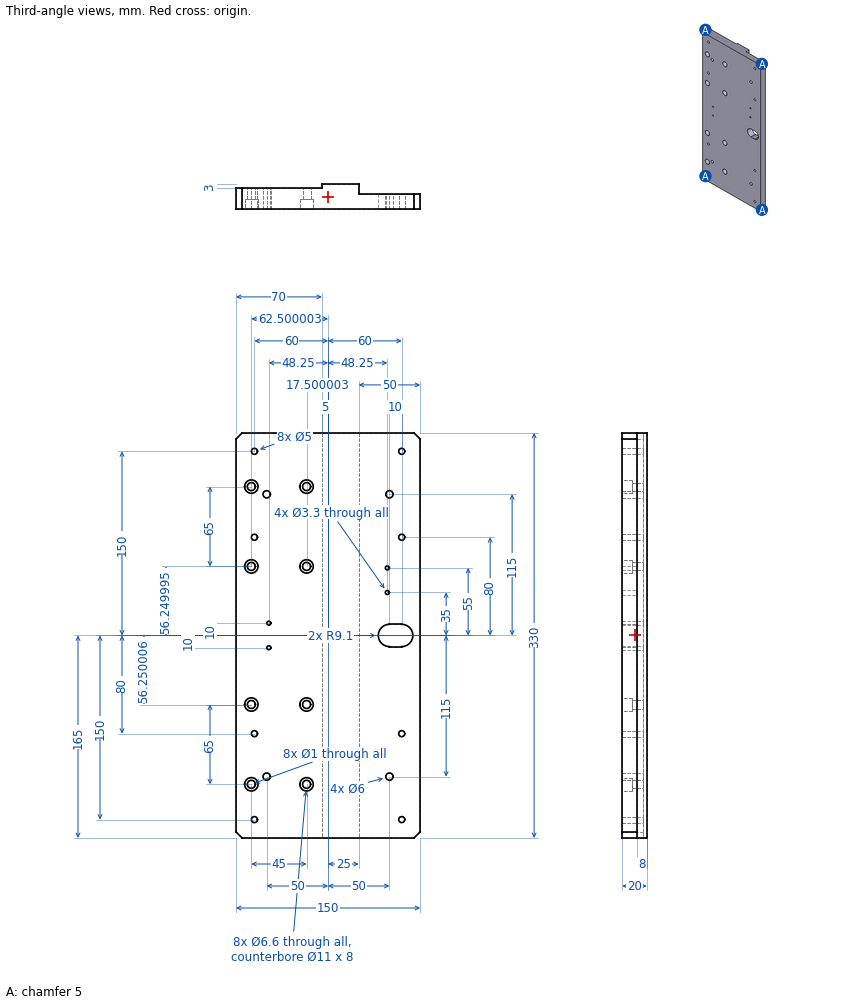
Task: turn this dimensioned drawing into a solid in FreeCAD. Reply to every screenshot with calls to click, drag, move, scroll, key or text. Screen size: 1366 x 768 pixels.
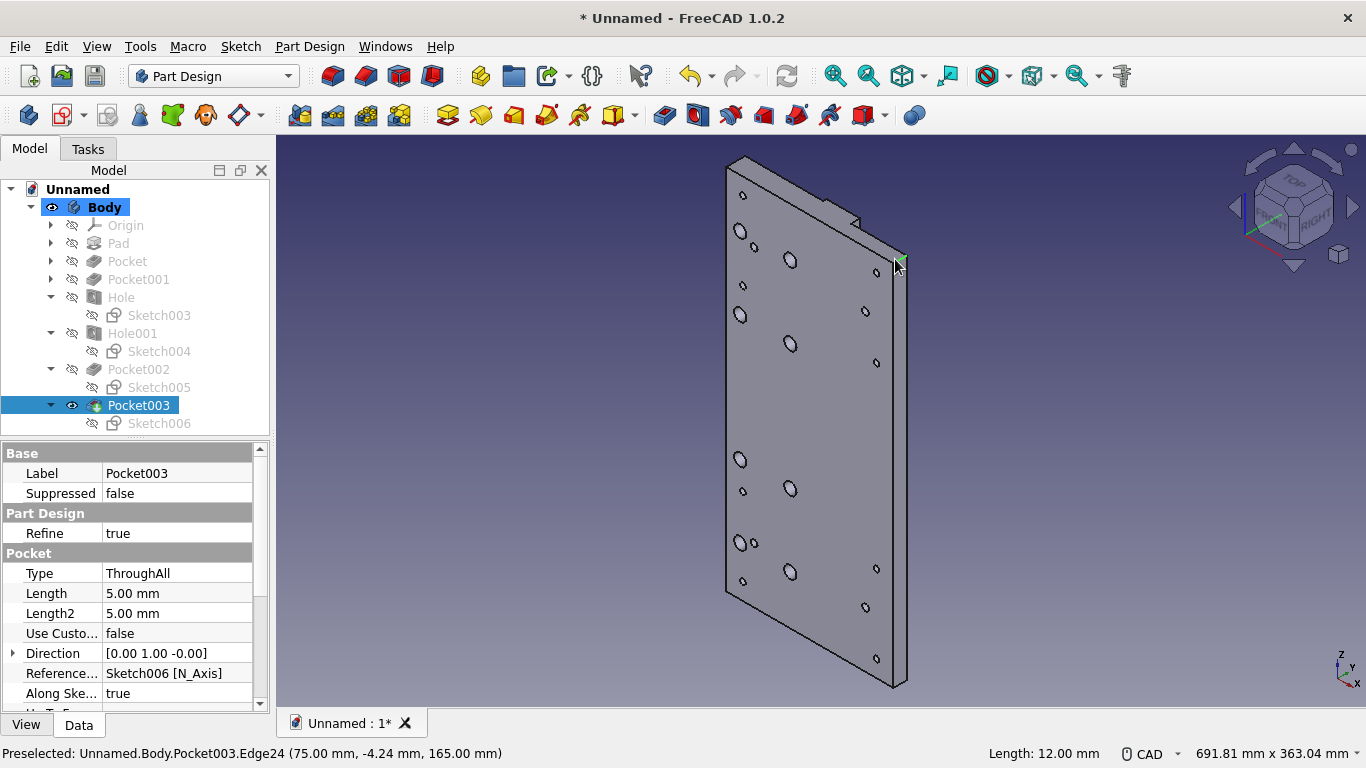
key(2)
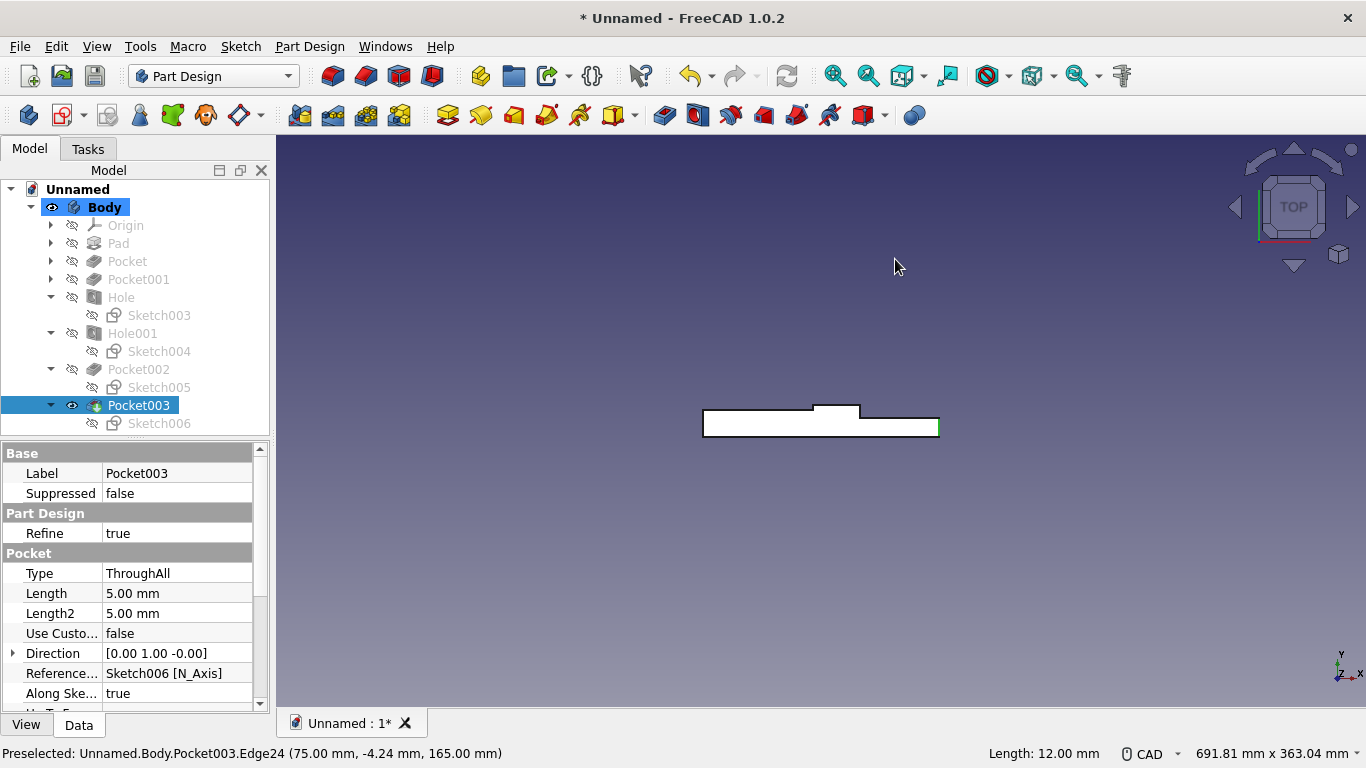
click(836, 76)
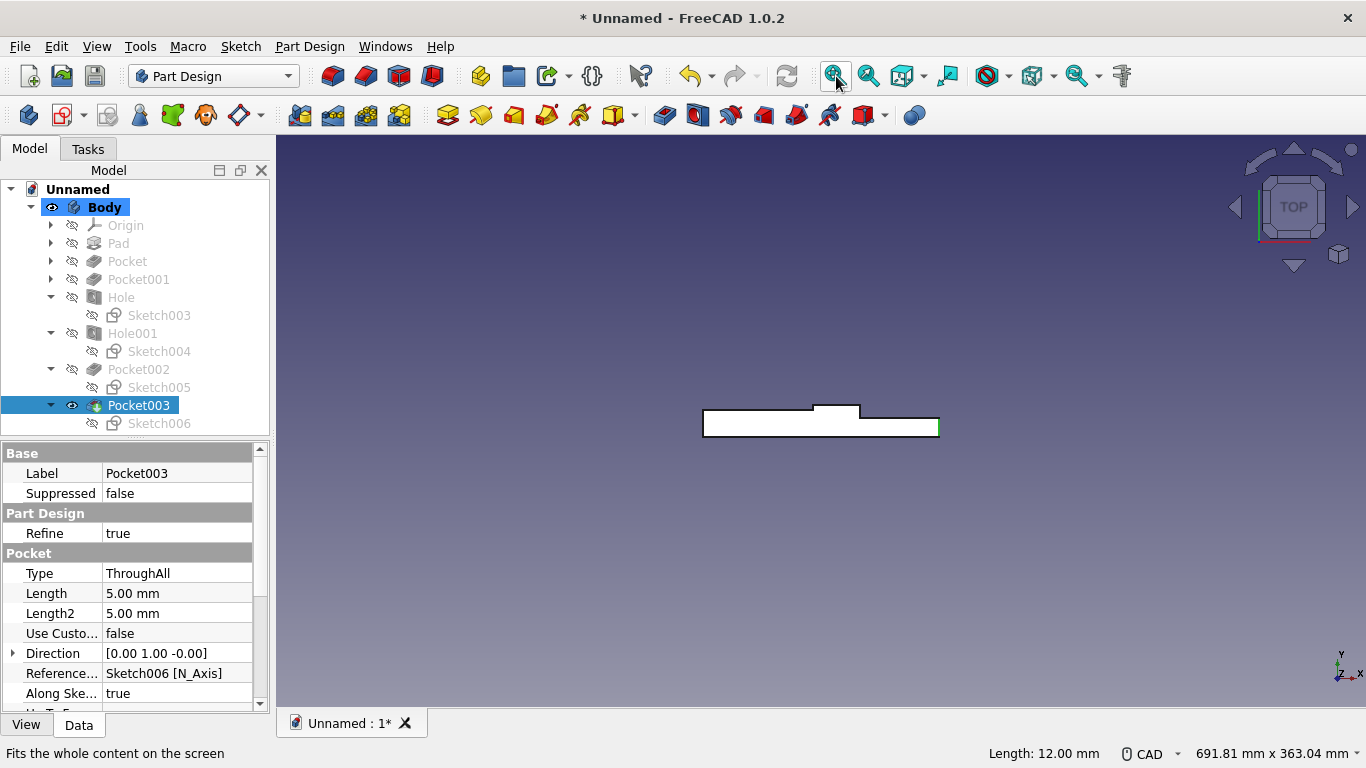
click(703, 422, ctrl)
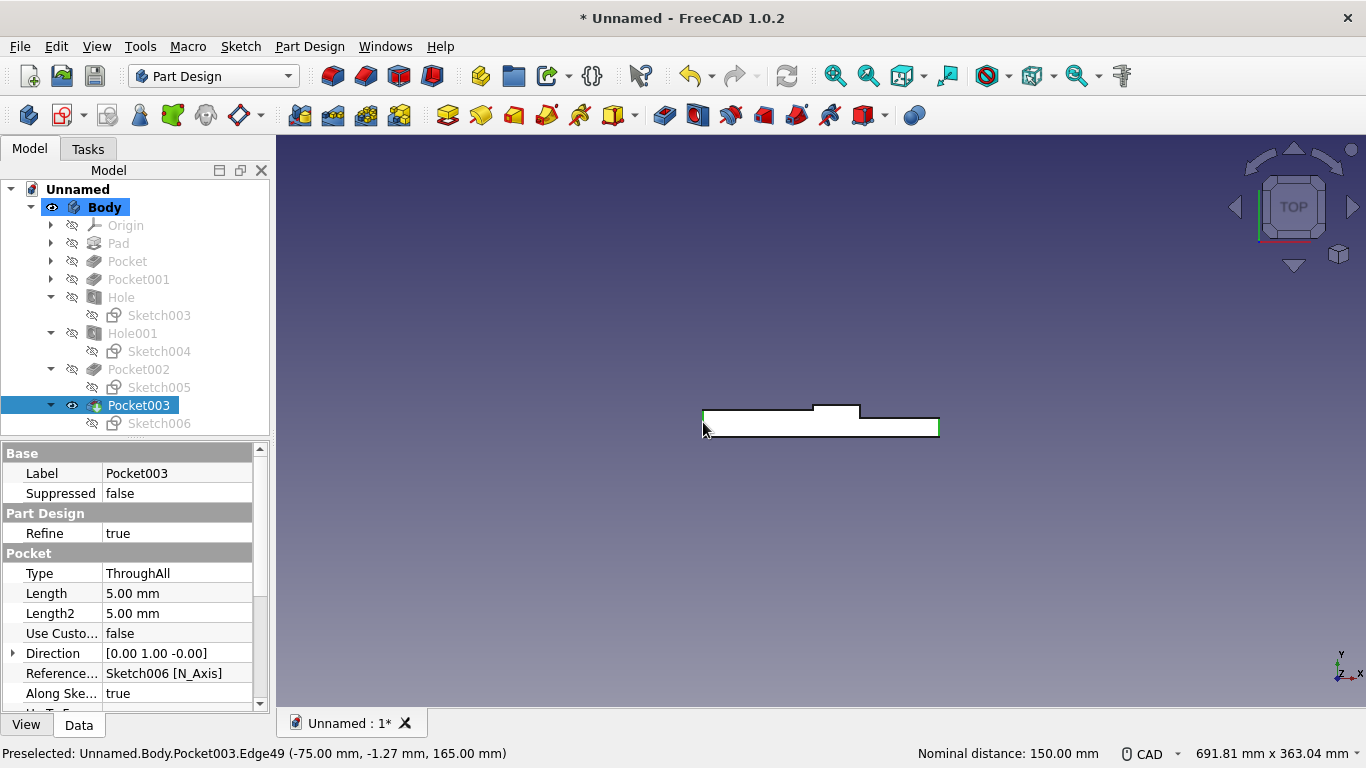
key(0)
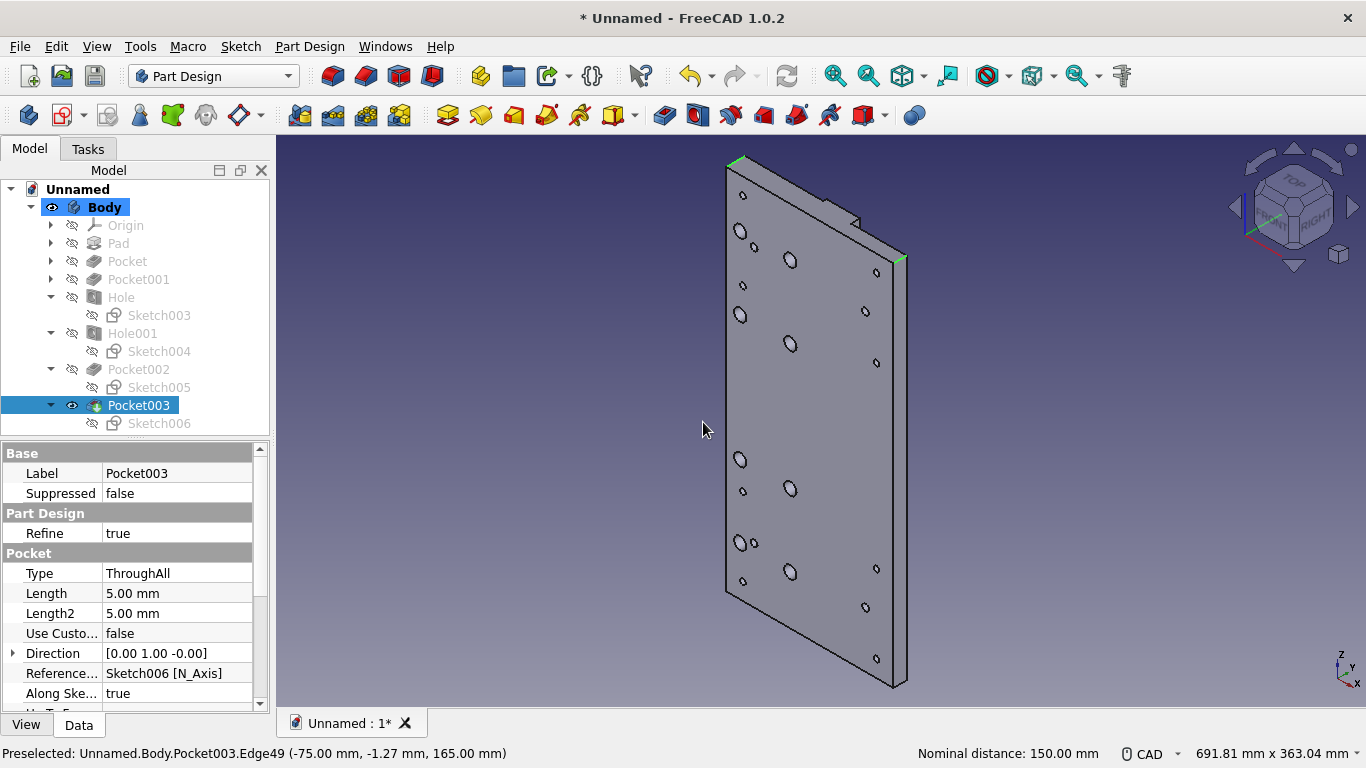
key(1)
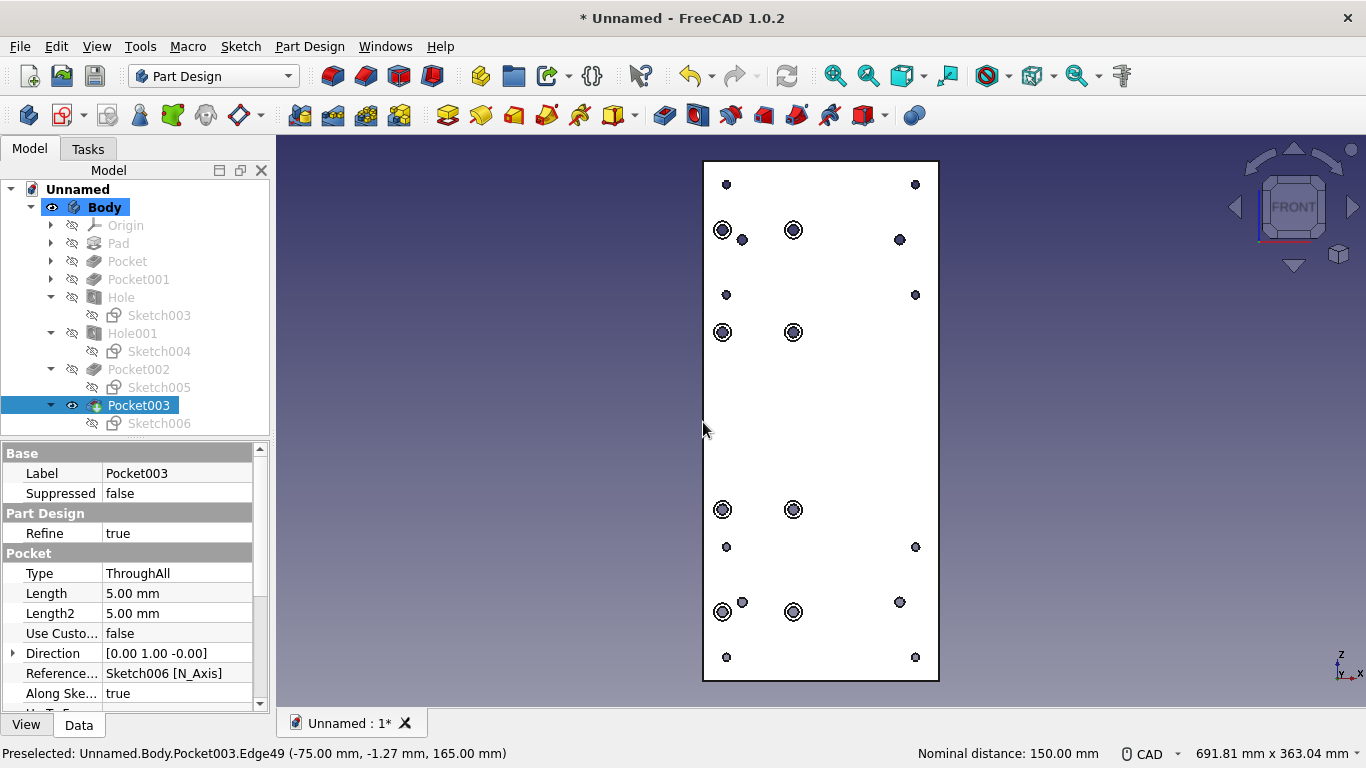
key(3)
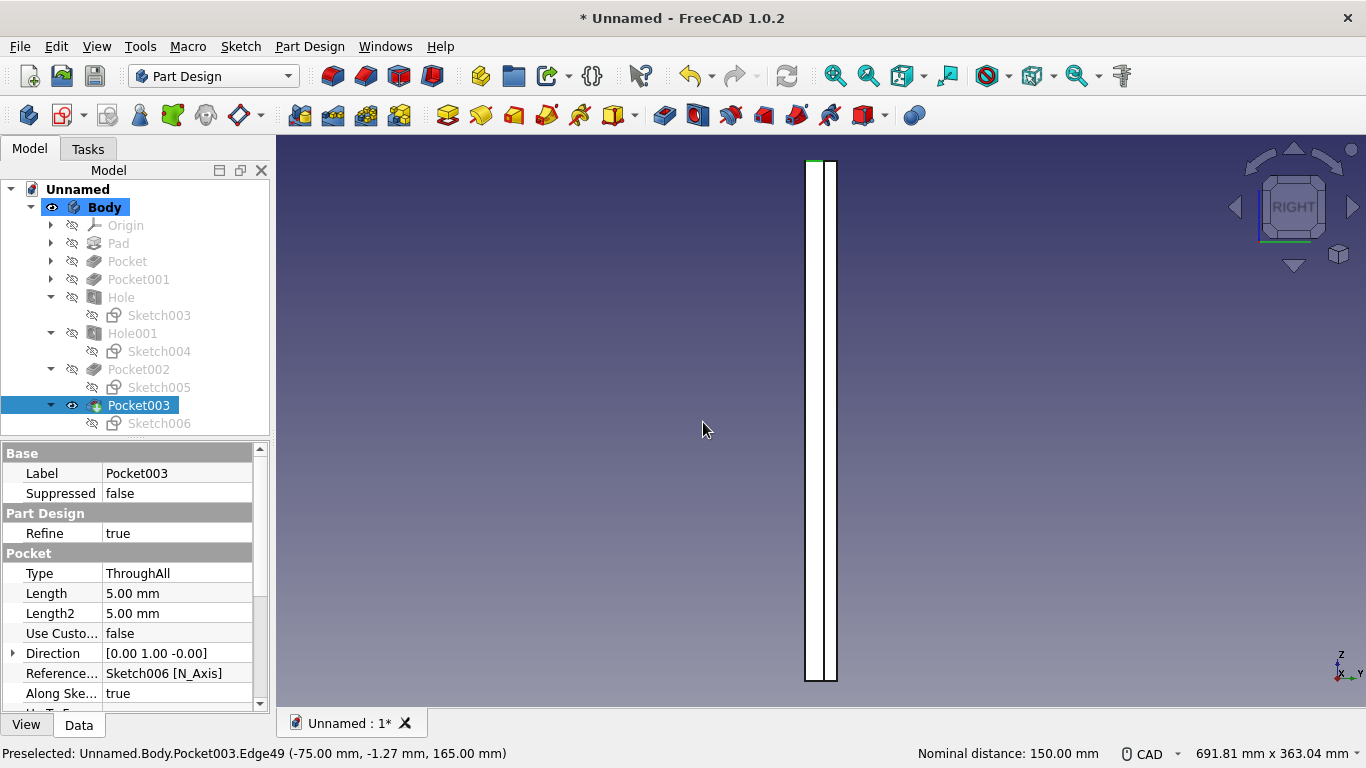
key(5)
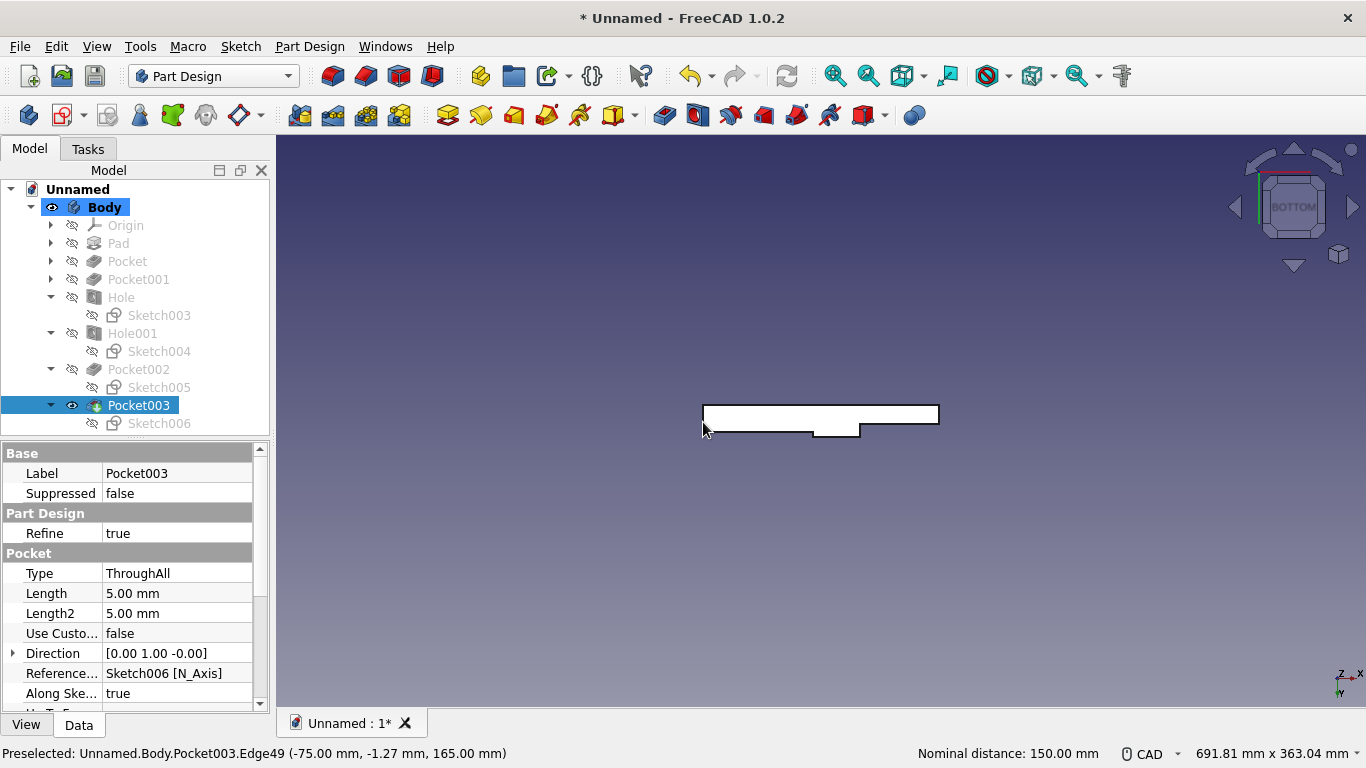
click(836, 76)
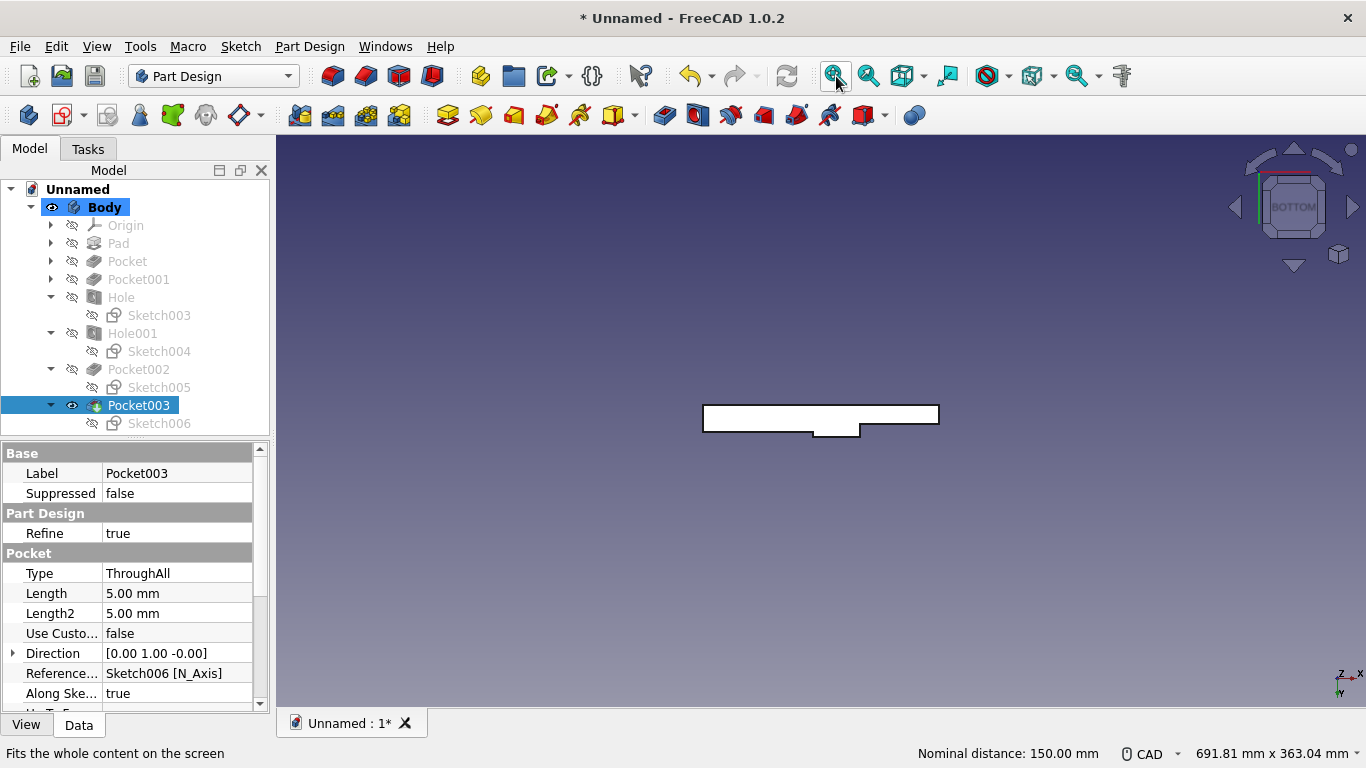
click(703, 418, ctrl)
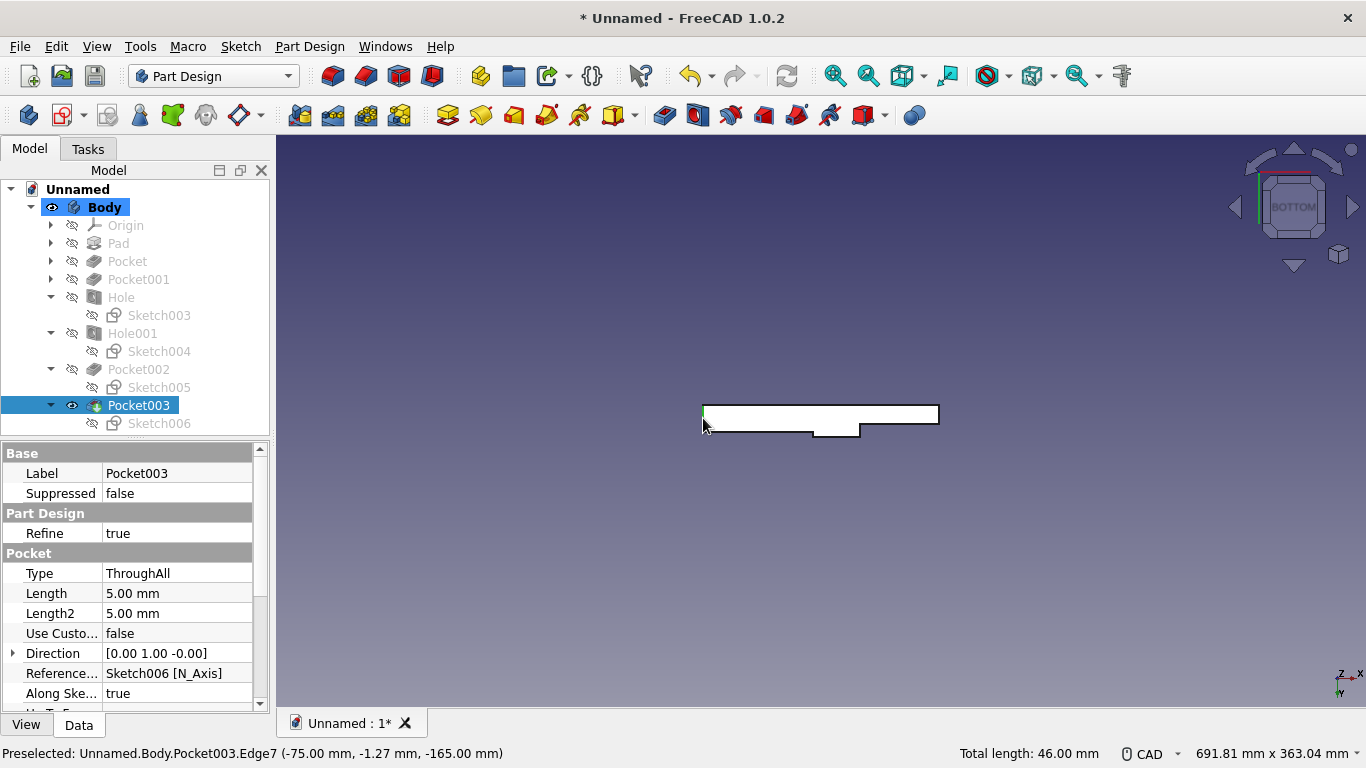
click(939, 414, ctrl)